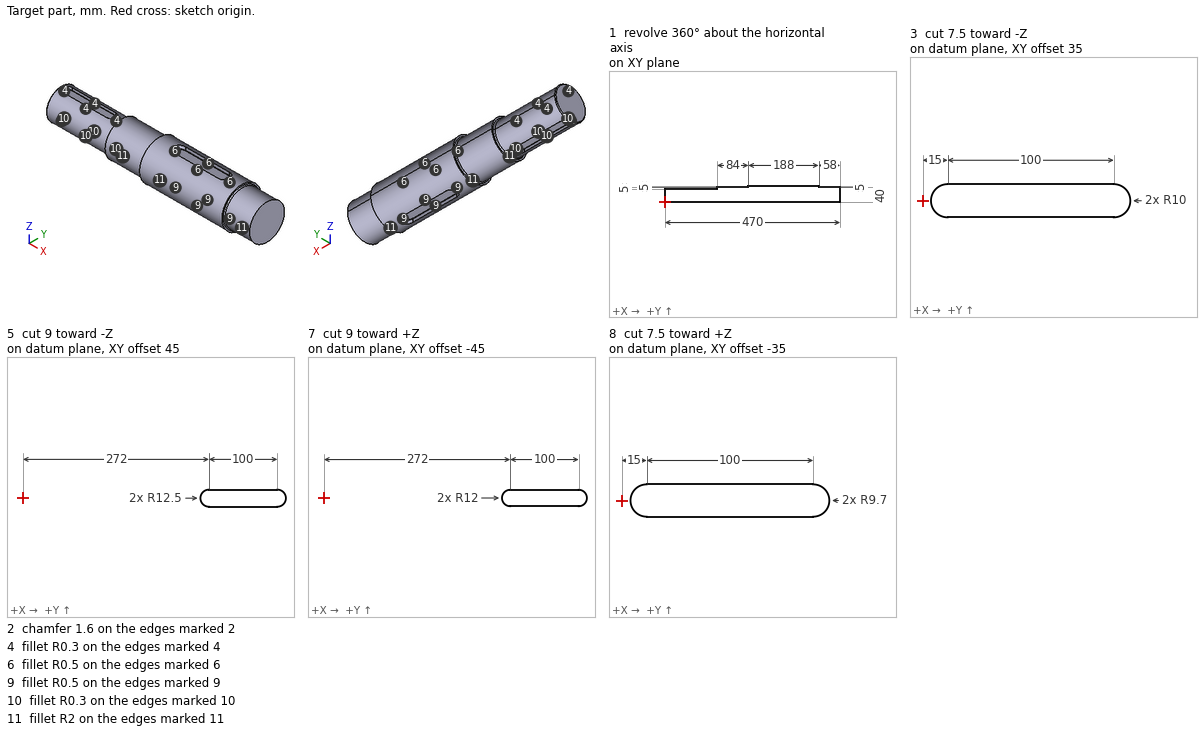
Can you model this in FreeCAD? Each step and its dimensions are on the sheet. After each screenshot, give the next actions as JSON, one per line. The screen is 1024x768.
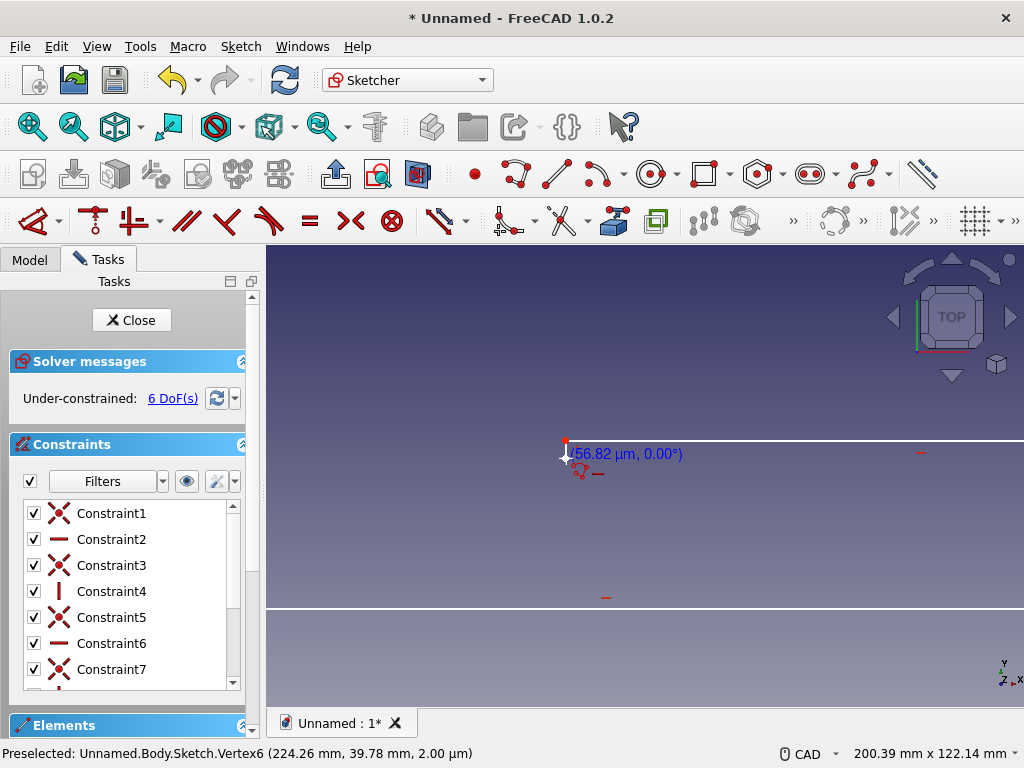
{"action": "scroll", "coordinate": [566, 460], "scroll_direction": "down", "scroll_amount": 7}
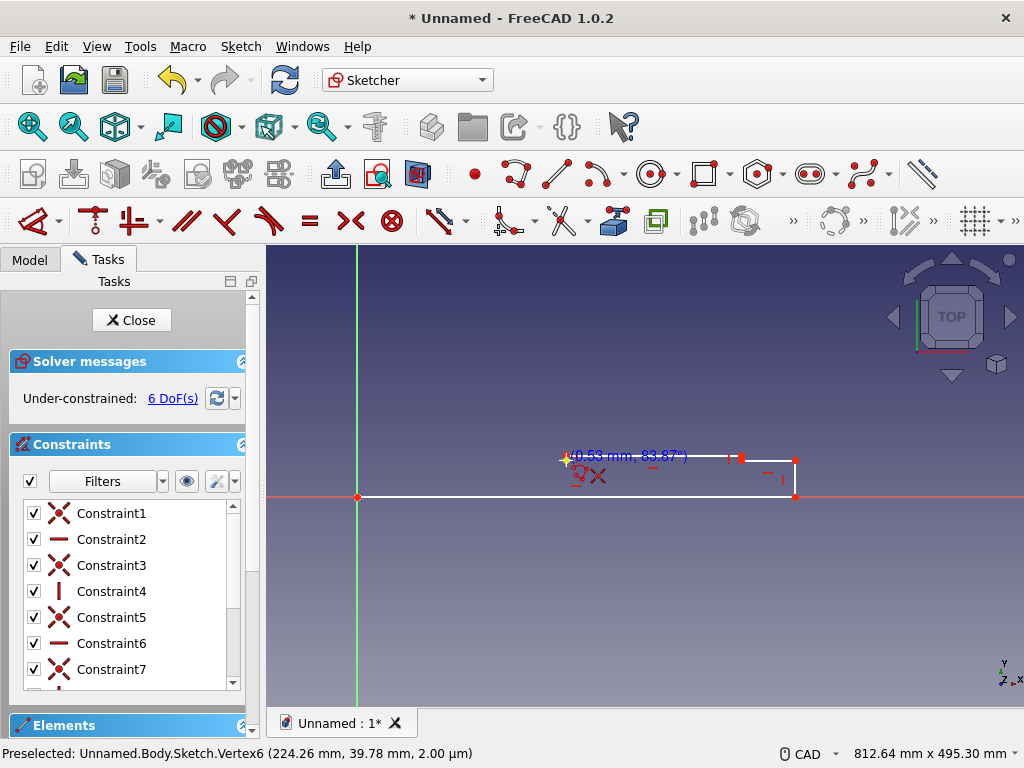
{"action": "left_click", "coordinate": [488, 460]}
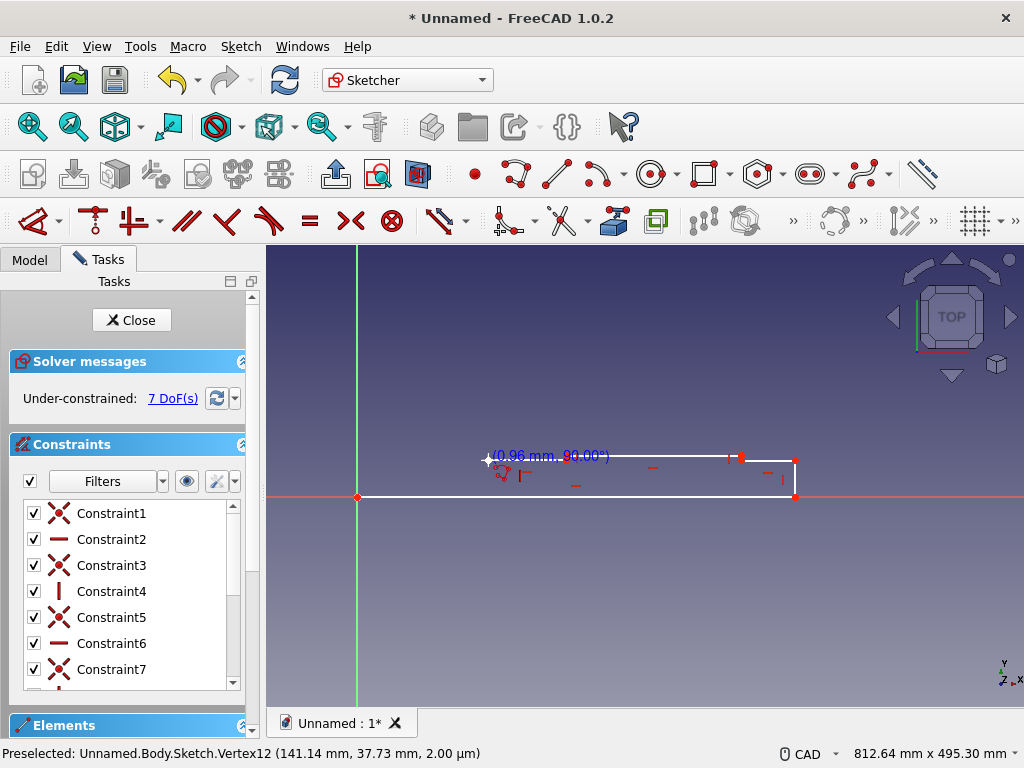
{"action": "scroll", "coordinate": [488, 465], "scroll_direction": "up", "scroll_amount": 7}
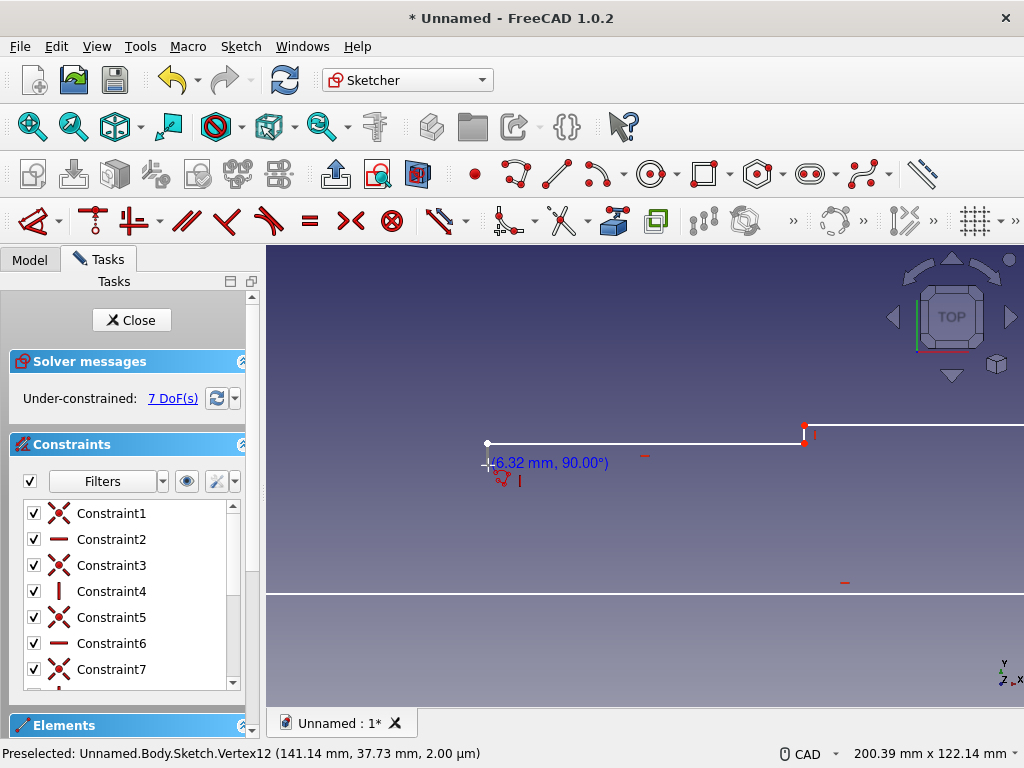
{"action": "left_click", "coordinate": [487, 462]}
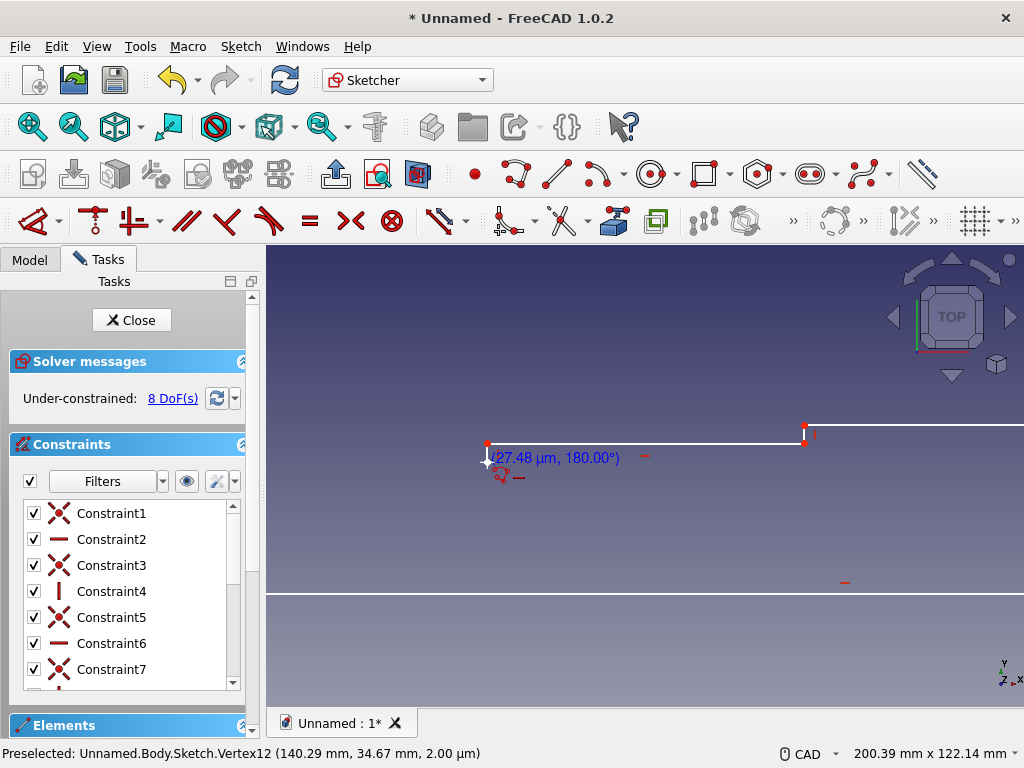
{"action": "scroll", "coordinate": [488, 465], "scroll_direction": "down", "scroll_amount": 7}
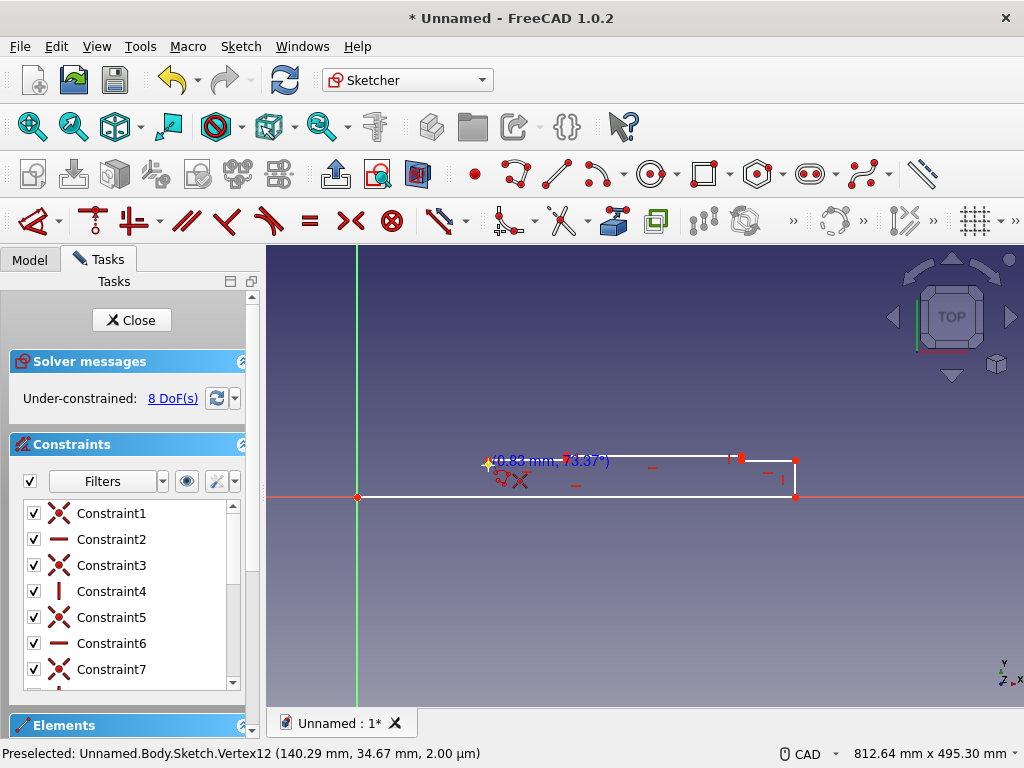
{"action": "left_click", "coordinate": [366, 465]}
{"action": "left_click", "coordinate": [357, 497]}
{"action": "key", "text": "Escape"}
{"action": "key", "text": "Escape"}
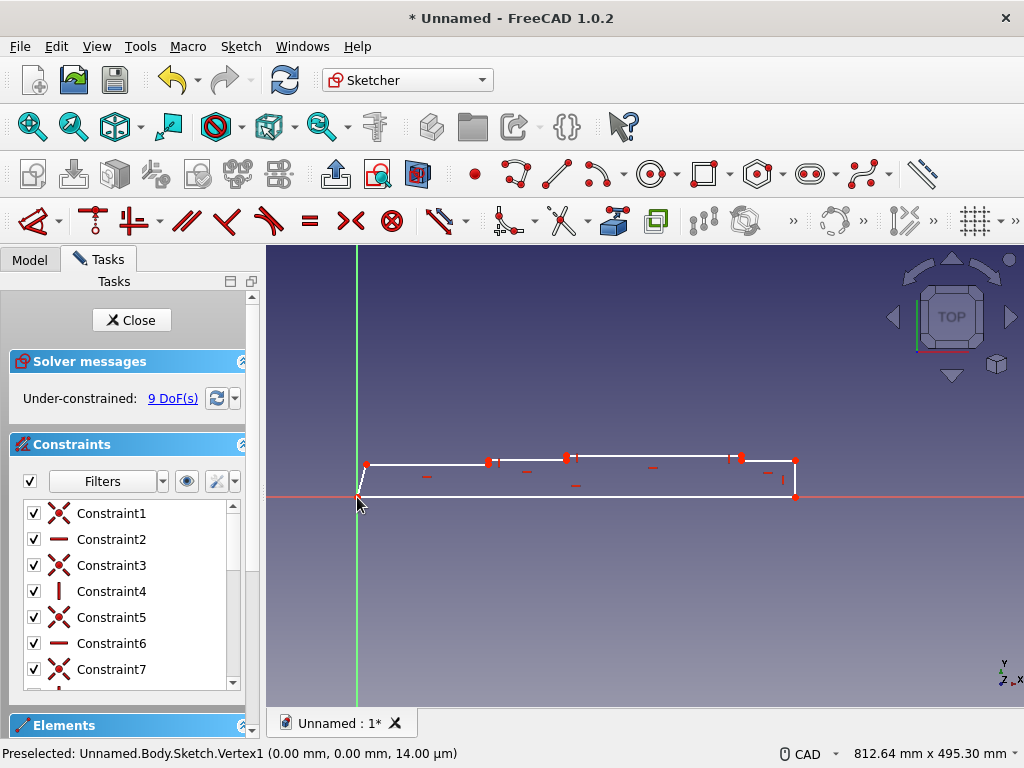
{"action": "scroll", "coordinate": [360, 487], "scroll_direction": "up", "scroll_amount": 2}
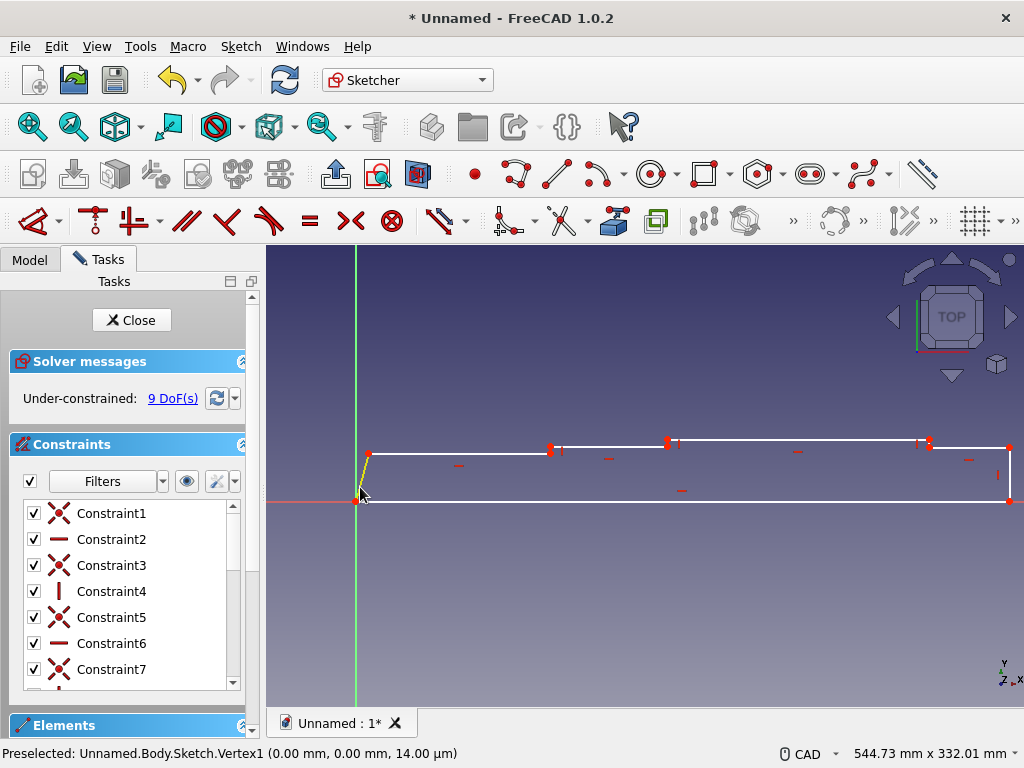
{"action": "left_click", "coordinate": [360, 487]}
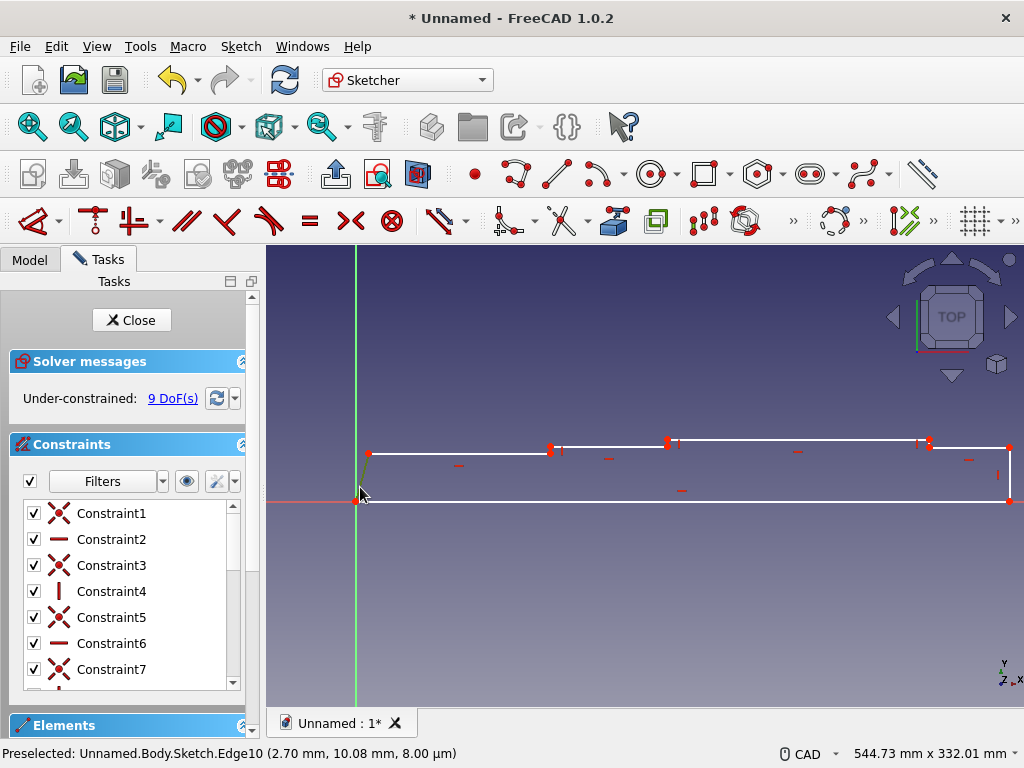
{"action": "left_click", "coordinate": [160, 222]}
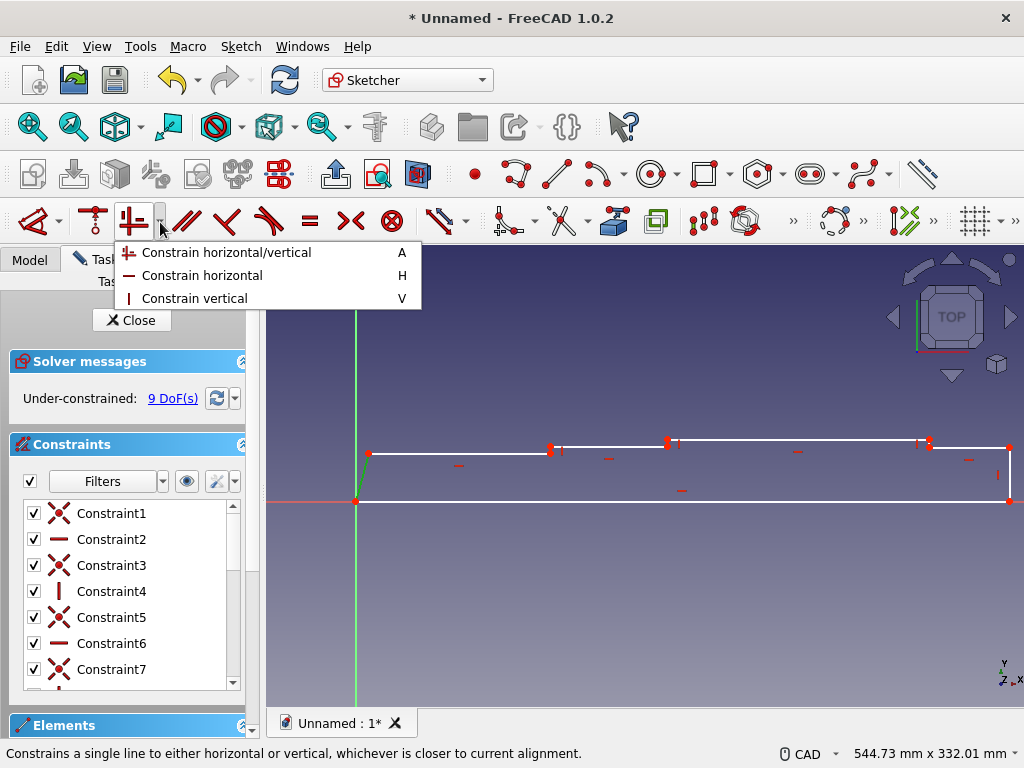
{"action": "left_click", "coordinate": [268, 298]}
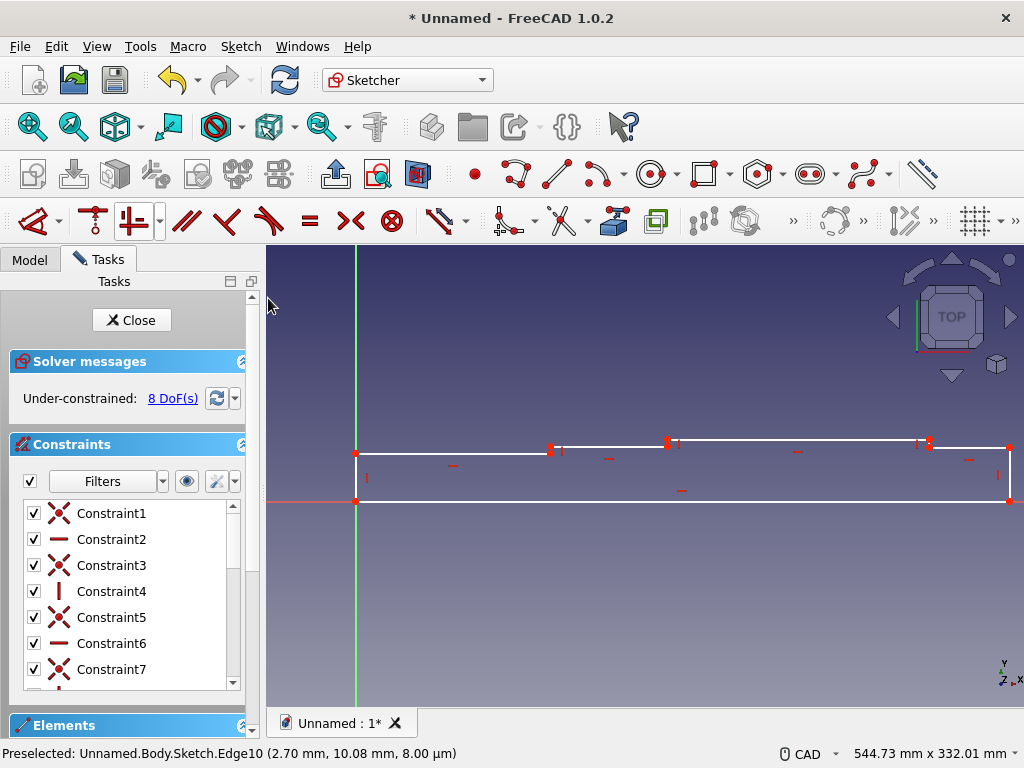
{"action": "scroll", "coordinate": [360, 487], "scroll_direction": "down", "scroll_amount": 2}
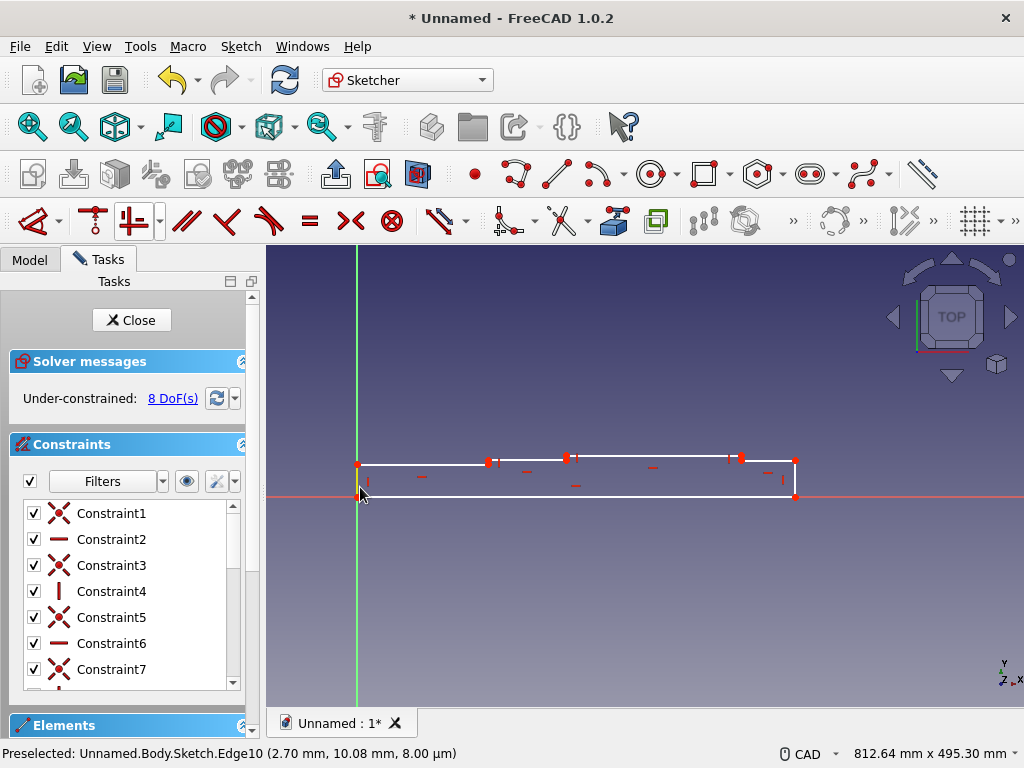
{"action": "scroll", "coordinate": [741, 458], "scroll_direction": "up", "scroll_amount": 11}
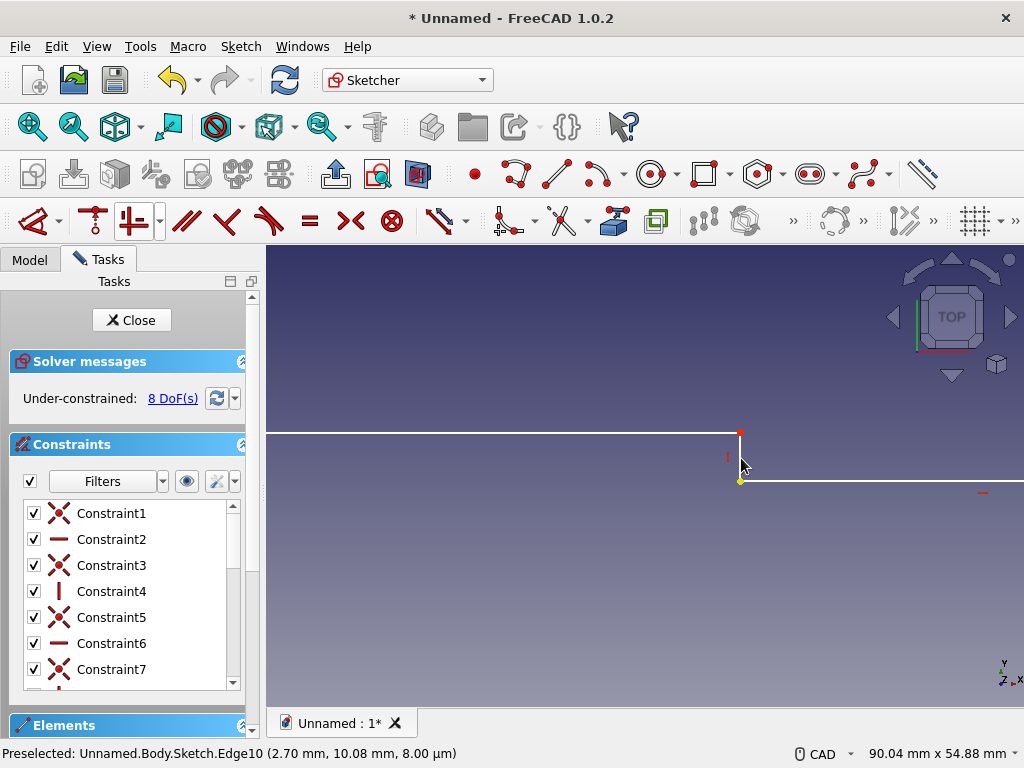
{"action": "left_click", "coordinate": [740, 457]}